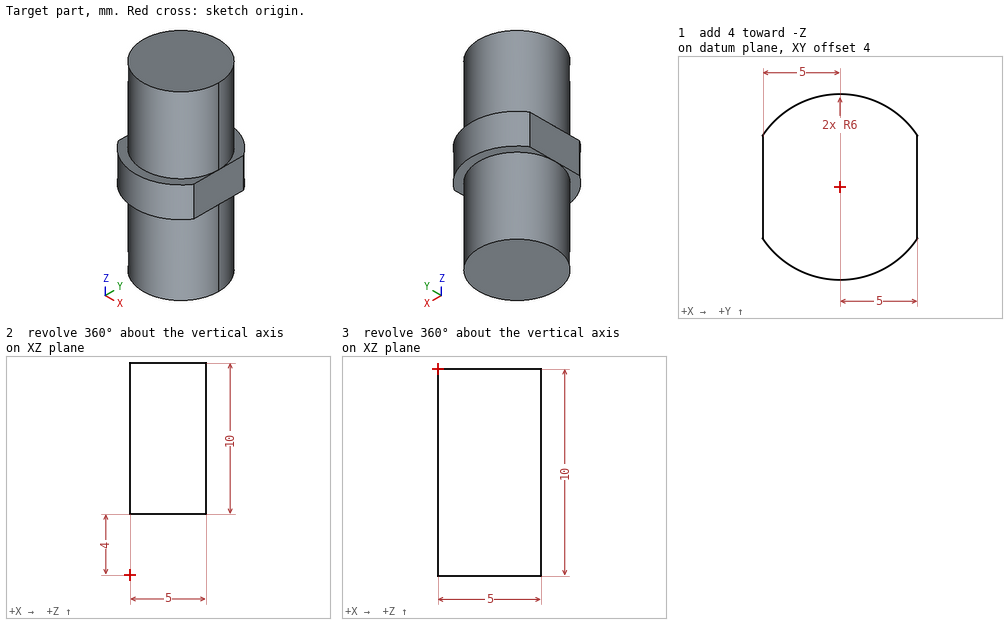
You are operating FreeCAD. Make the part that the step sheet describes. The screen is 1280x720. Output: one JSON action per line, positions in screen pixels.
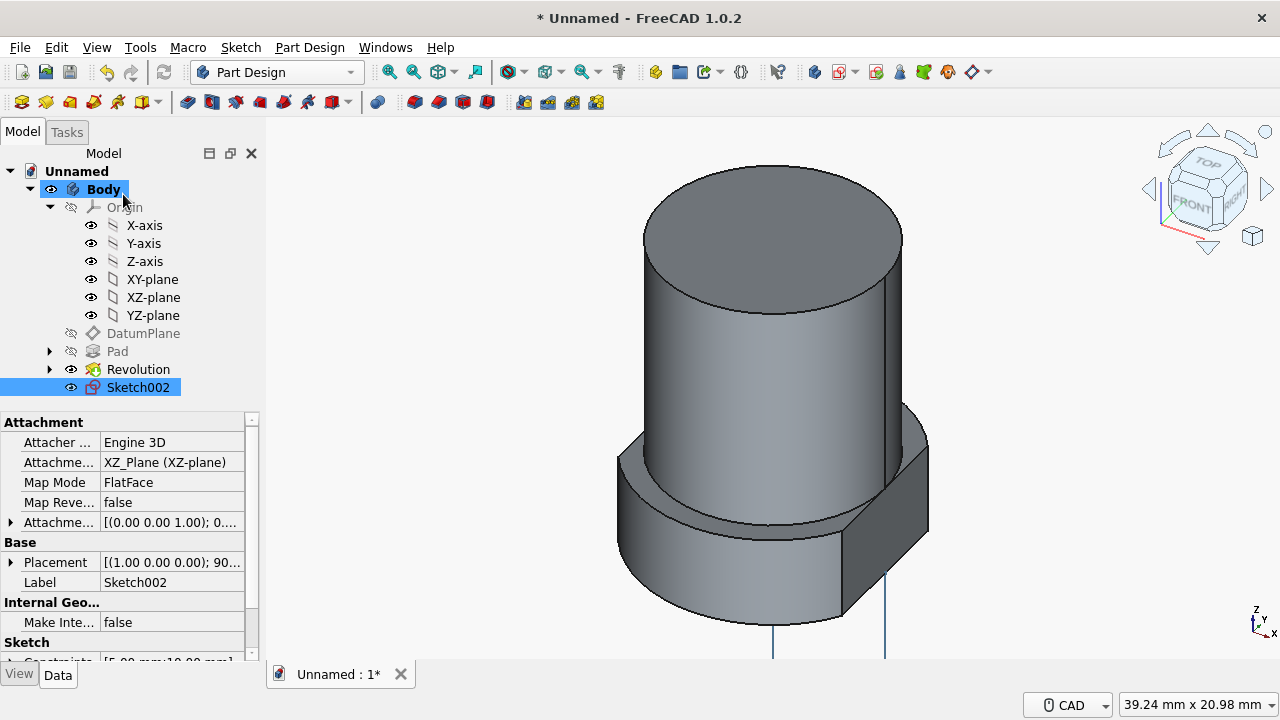
{"action": "left_click", "coordinate": [46, 102]}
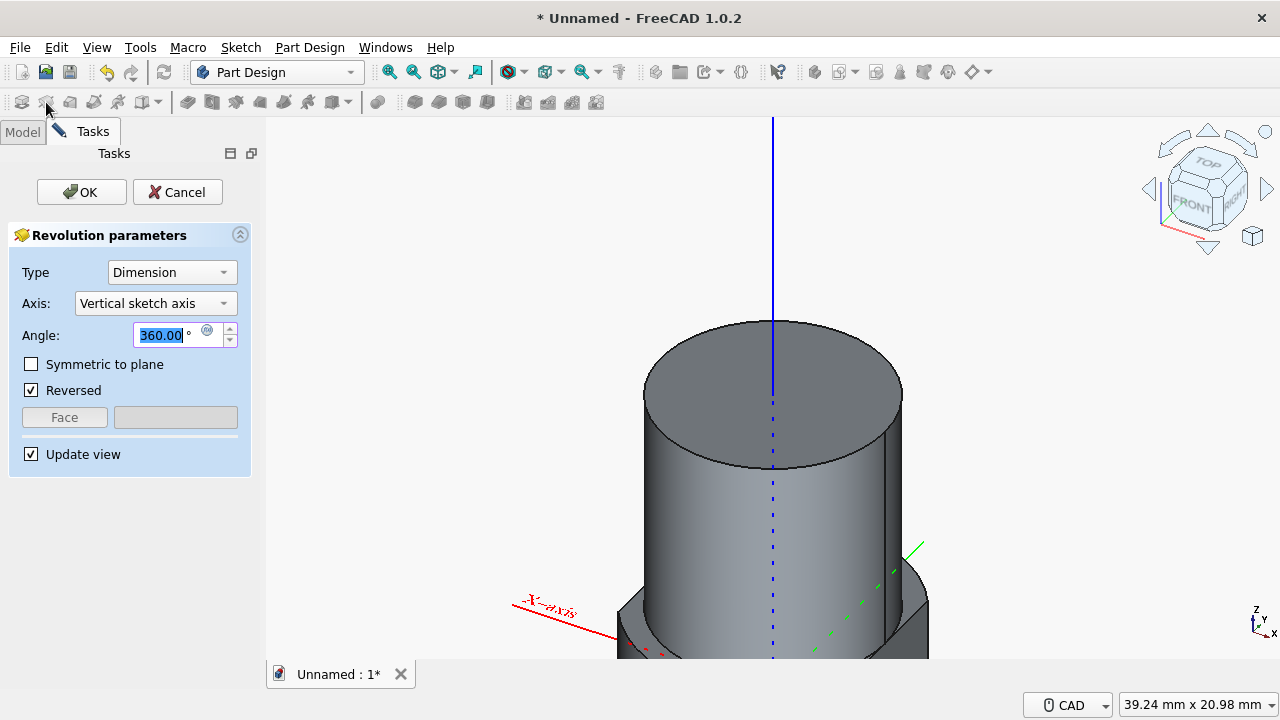
{"action": "left_click", "coordinate": [82, 192]}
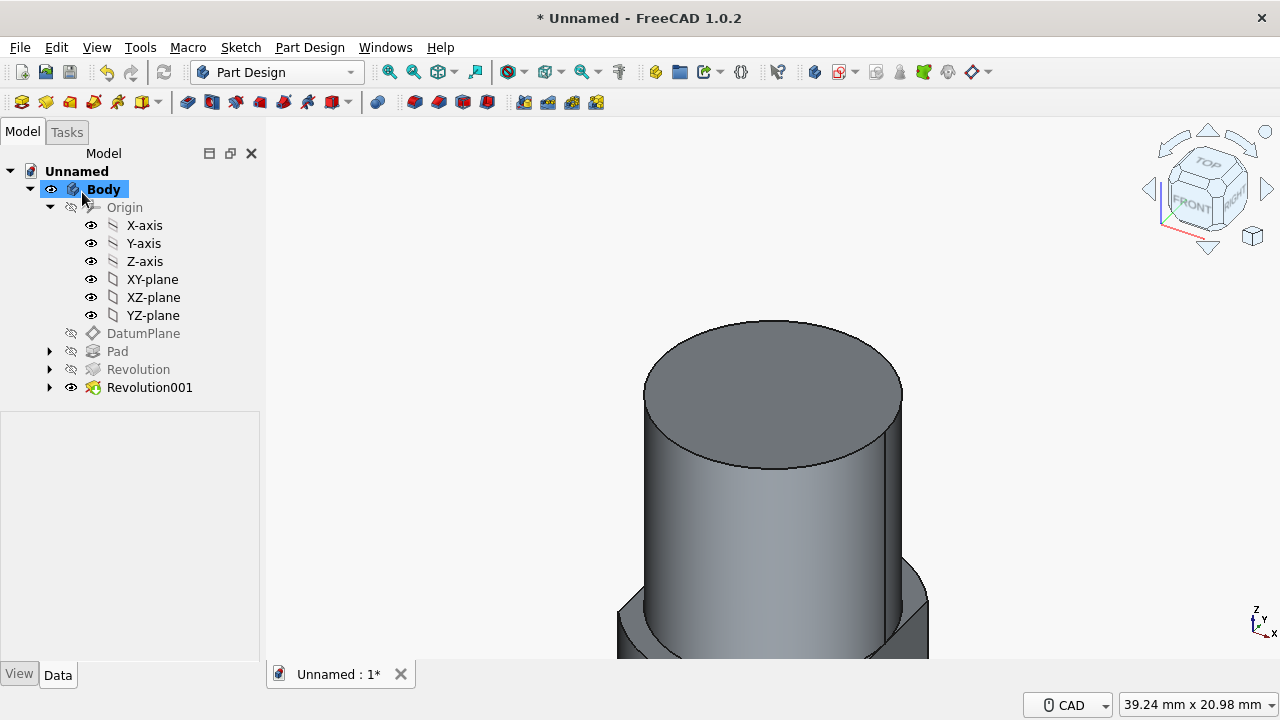
{"action": "key", "text": "0"}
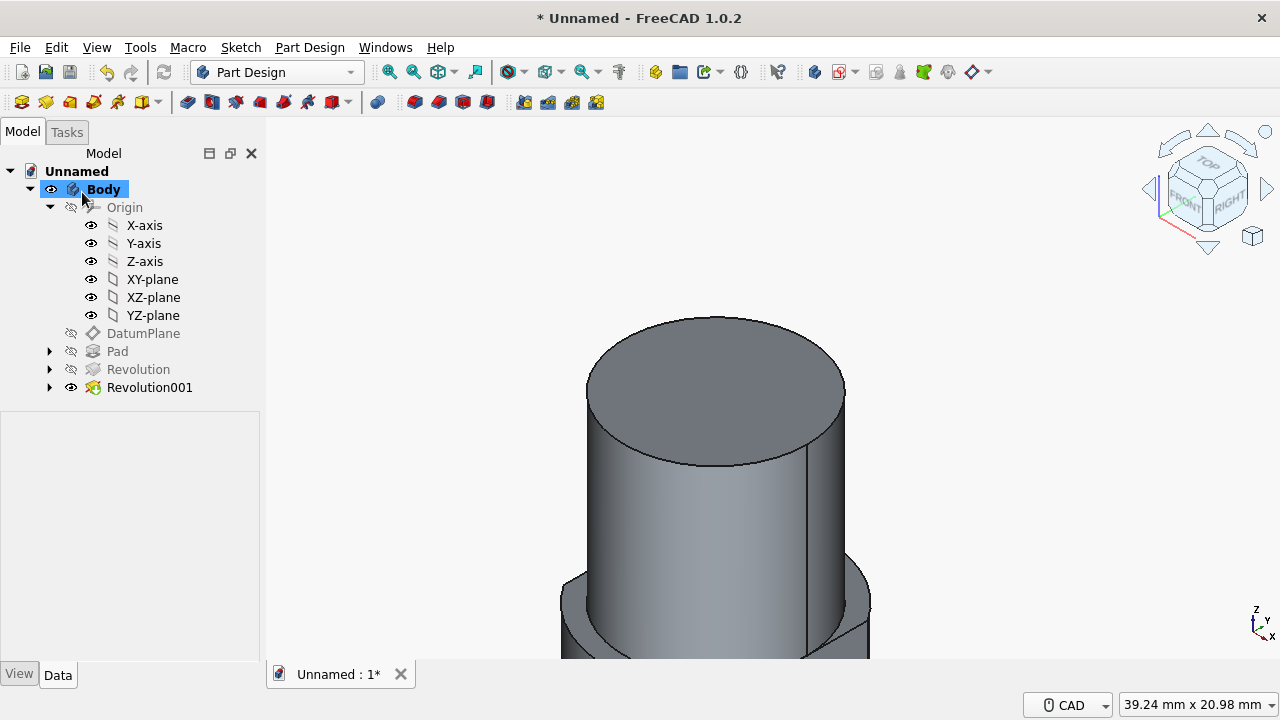
{"action": "left_click", "coordinate": [390, 72]}